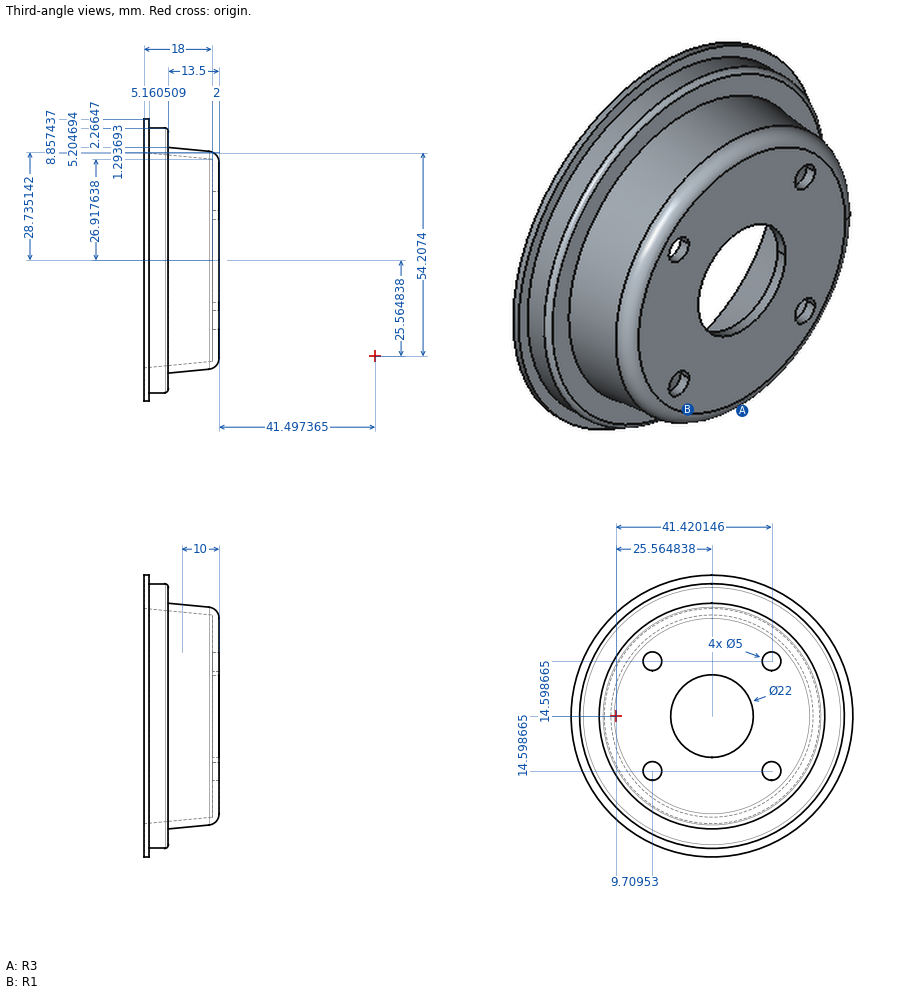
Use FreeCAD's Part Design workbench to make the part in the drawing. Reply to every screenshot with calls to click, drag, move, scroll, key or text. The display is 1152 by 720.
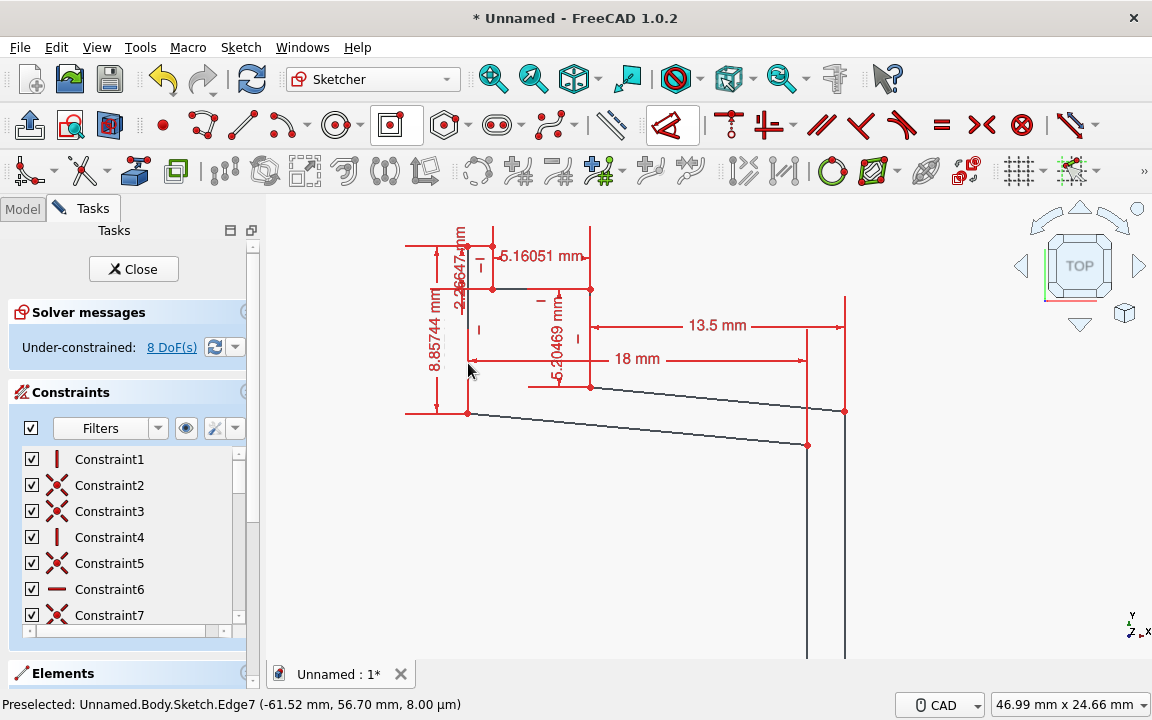
scroll(507, 292, down, 7)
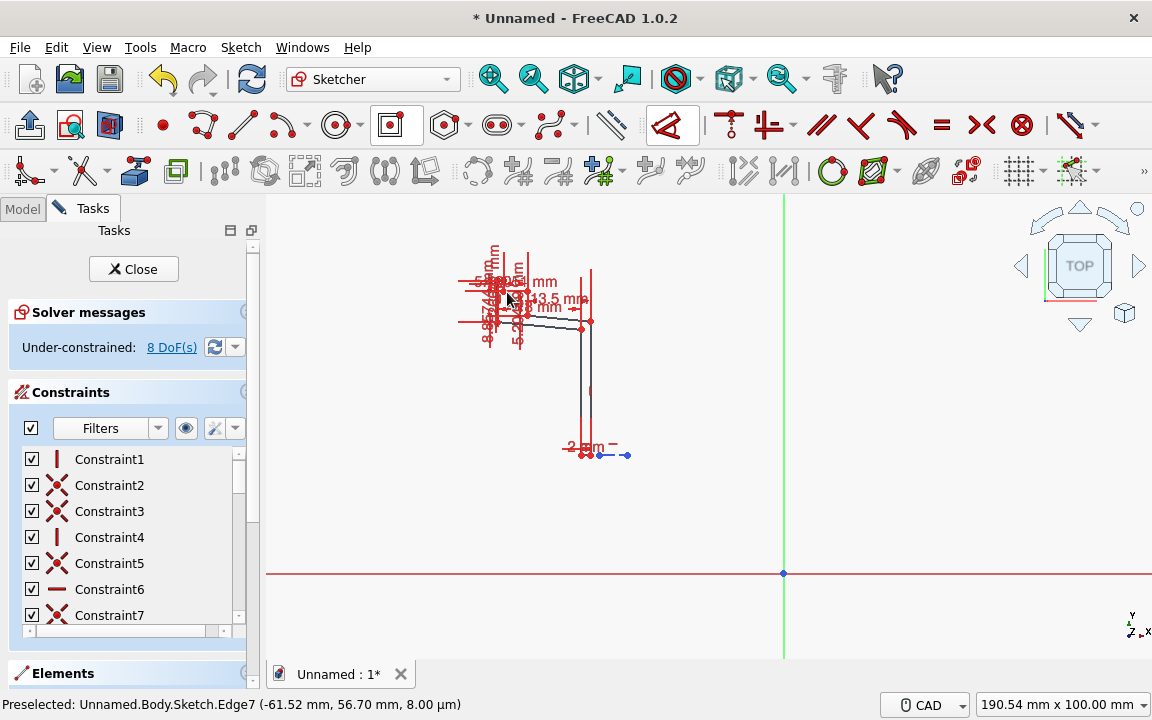
click(498, 322)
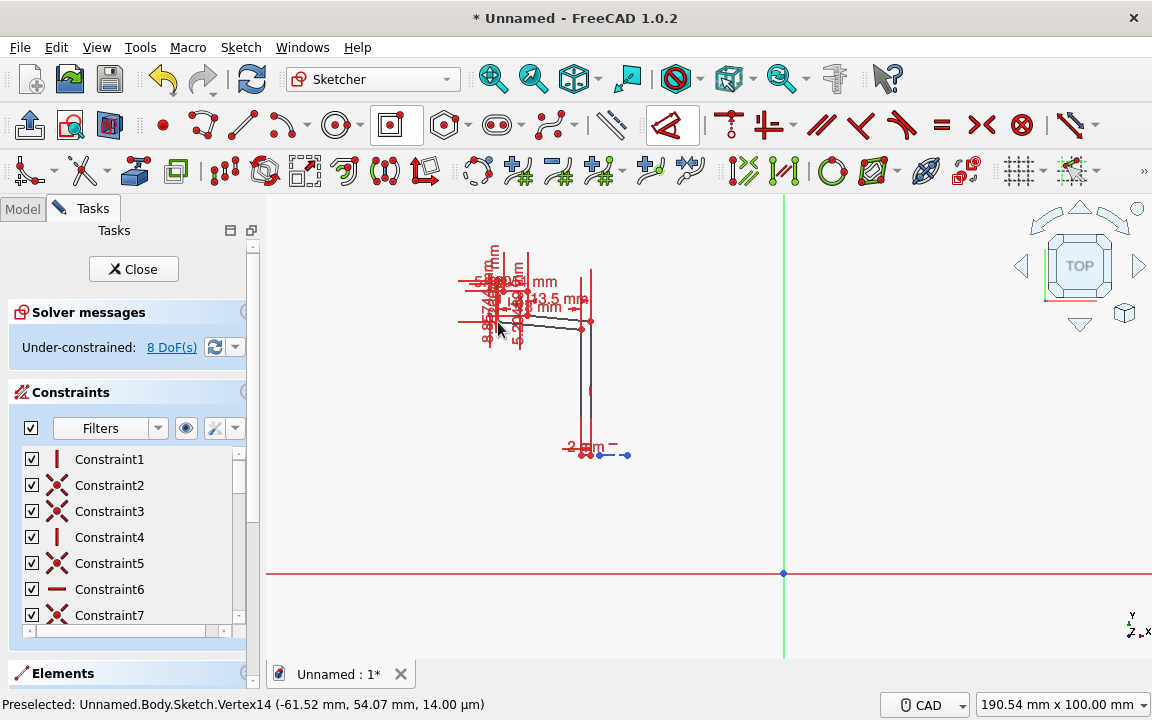
key(i)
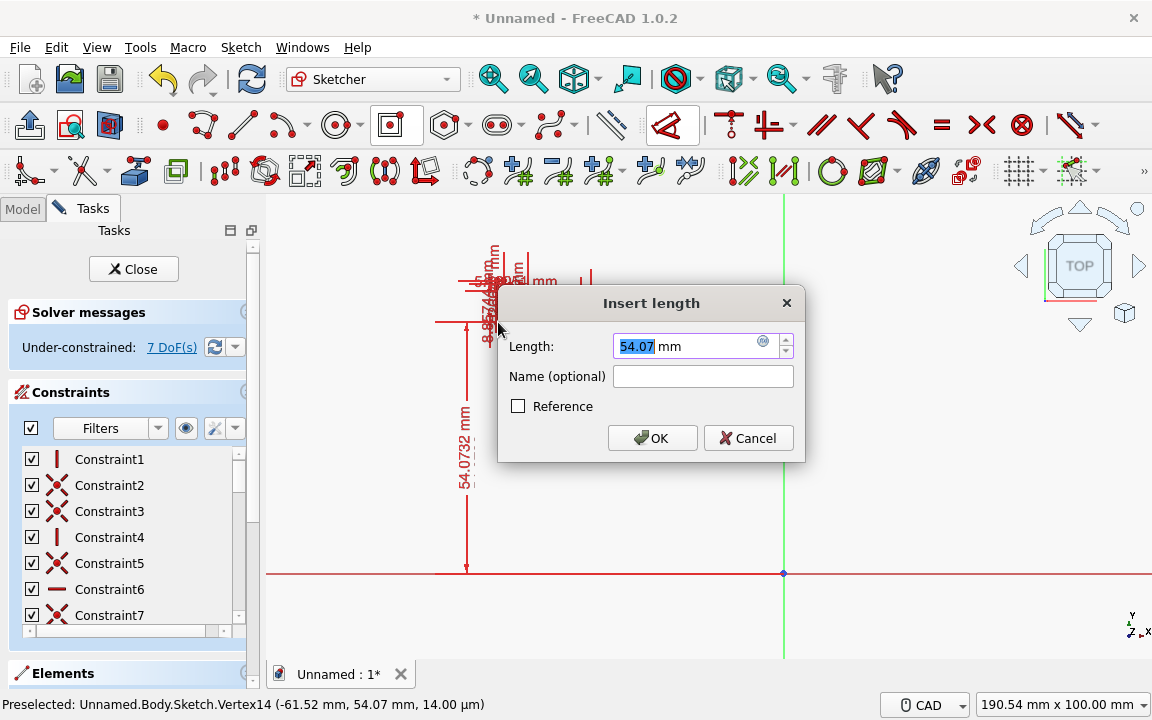
text(54.2074)
key(Return)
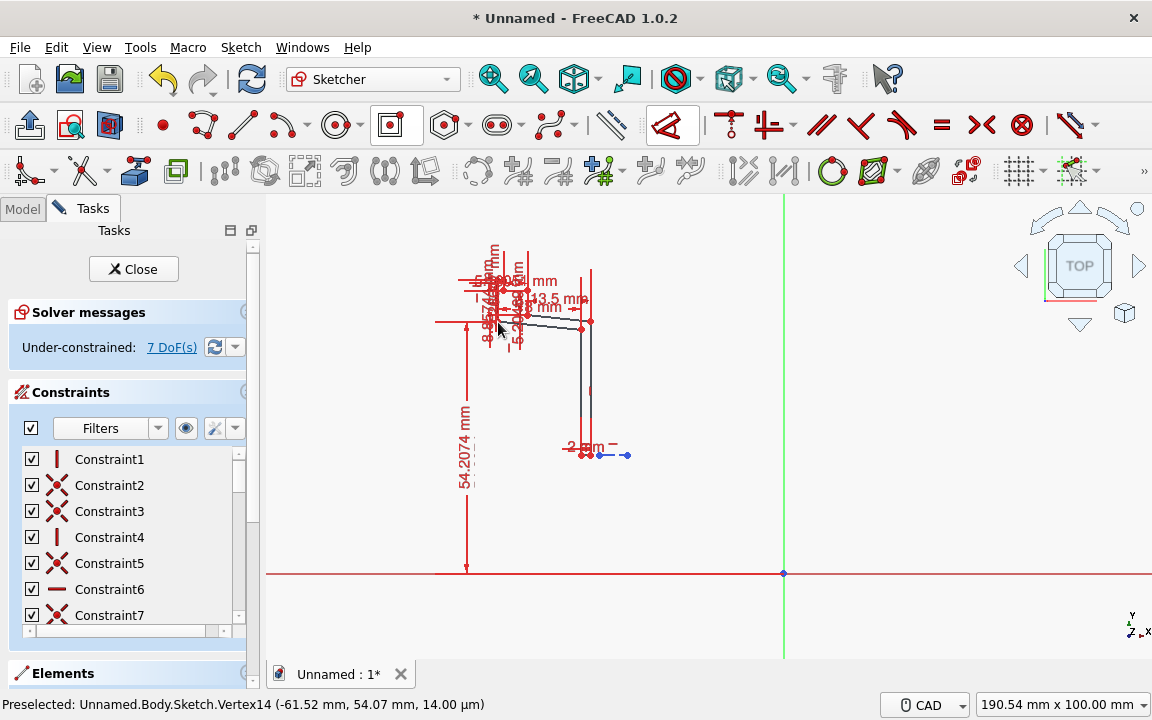
scroll(591, 415, up, 2)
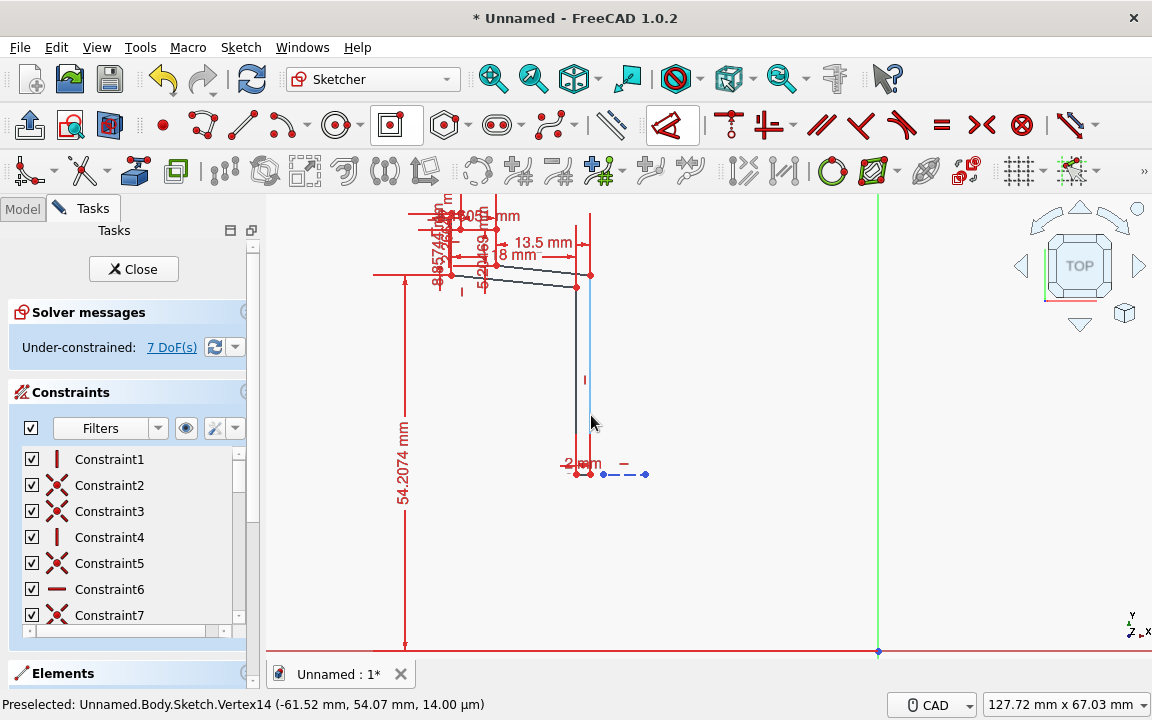
click(590, 415)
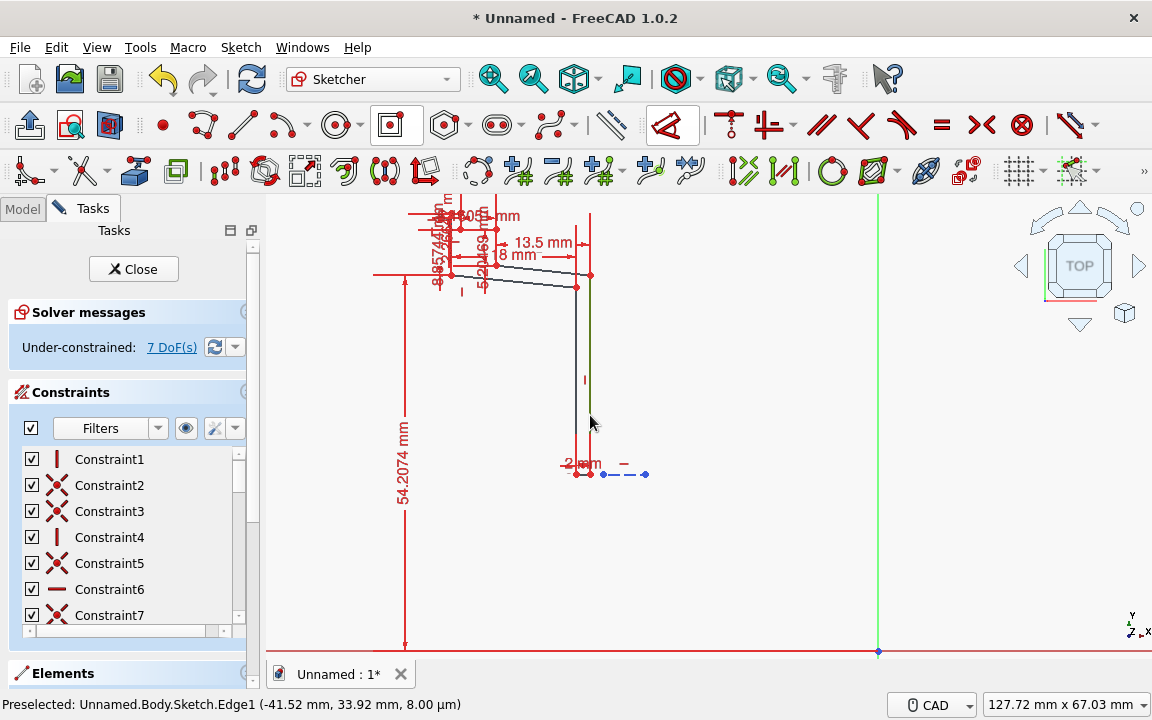
key(i)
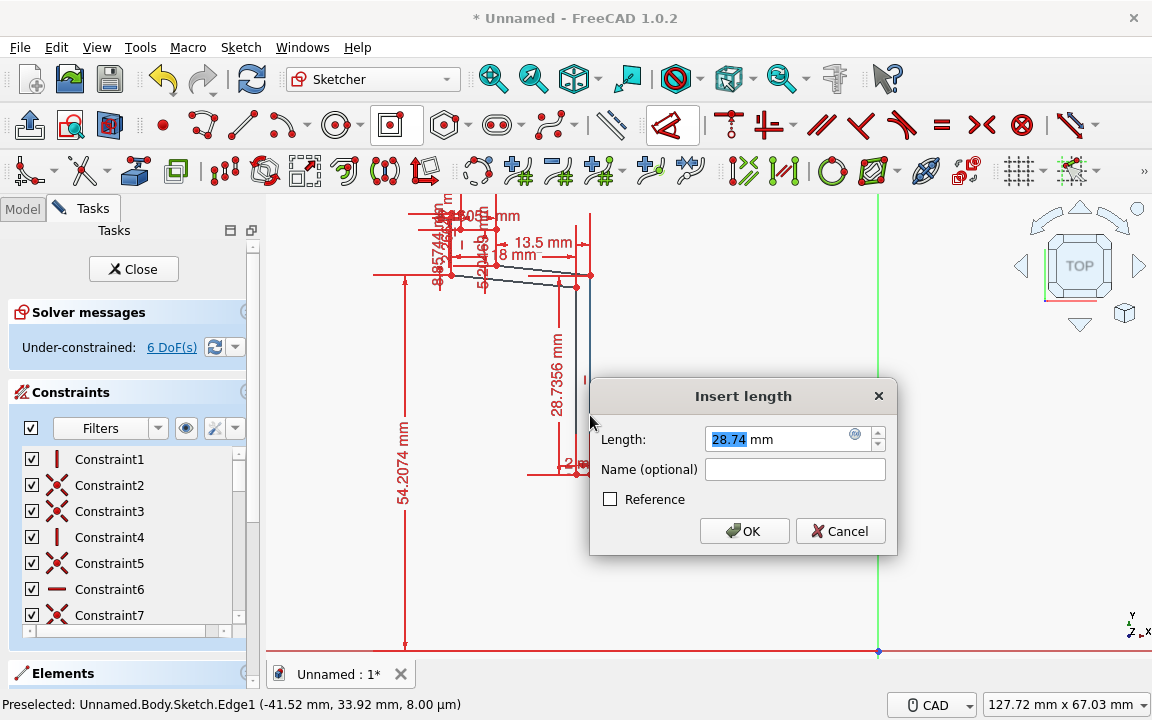
text(28.735142)
key(Return)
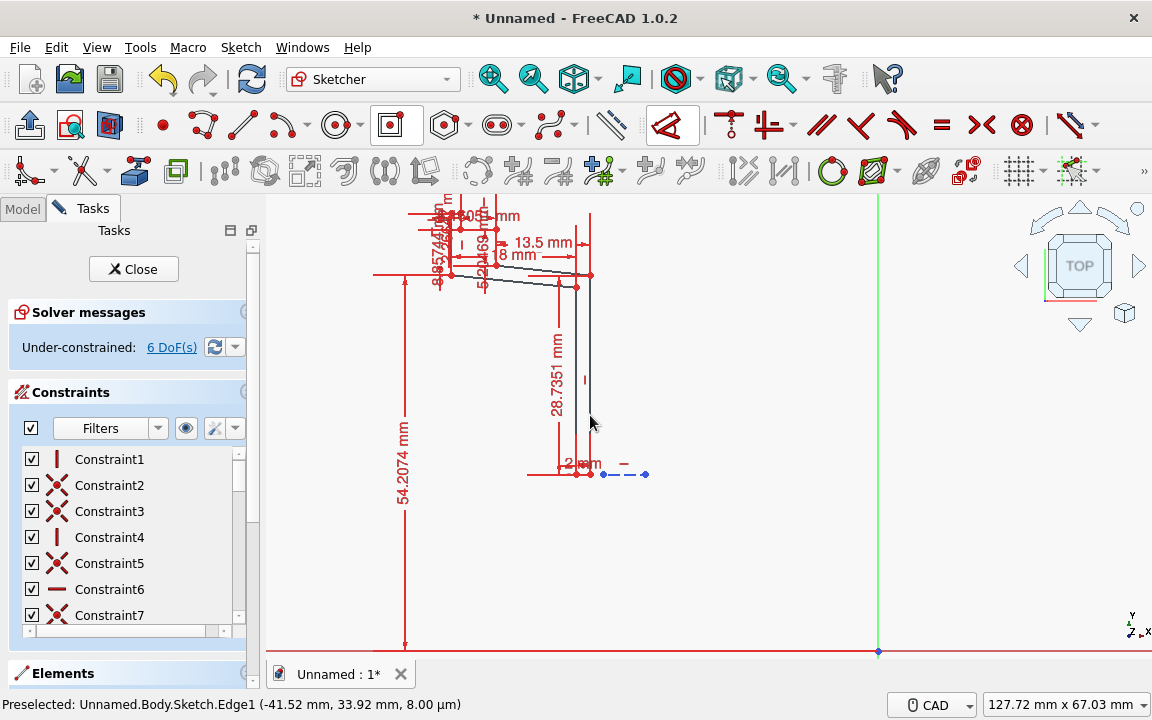
click(576, 344)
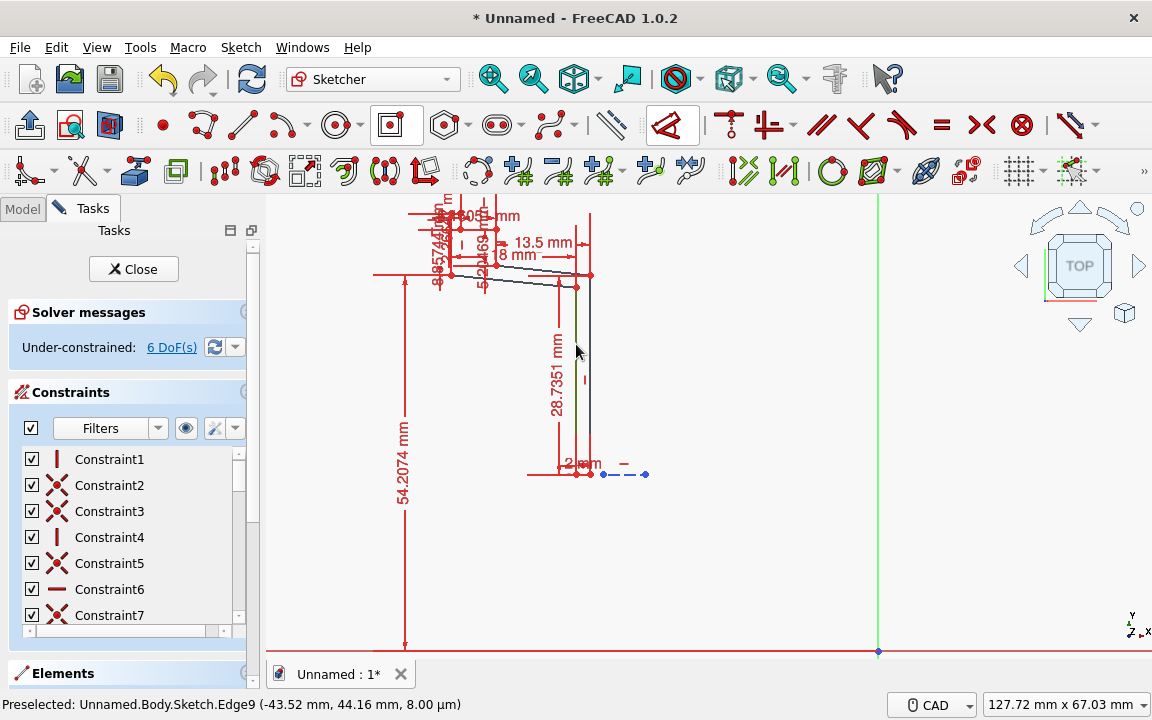
key(i)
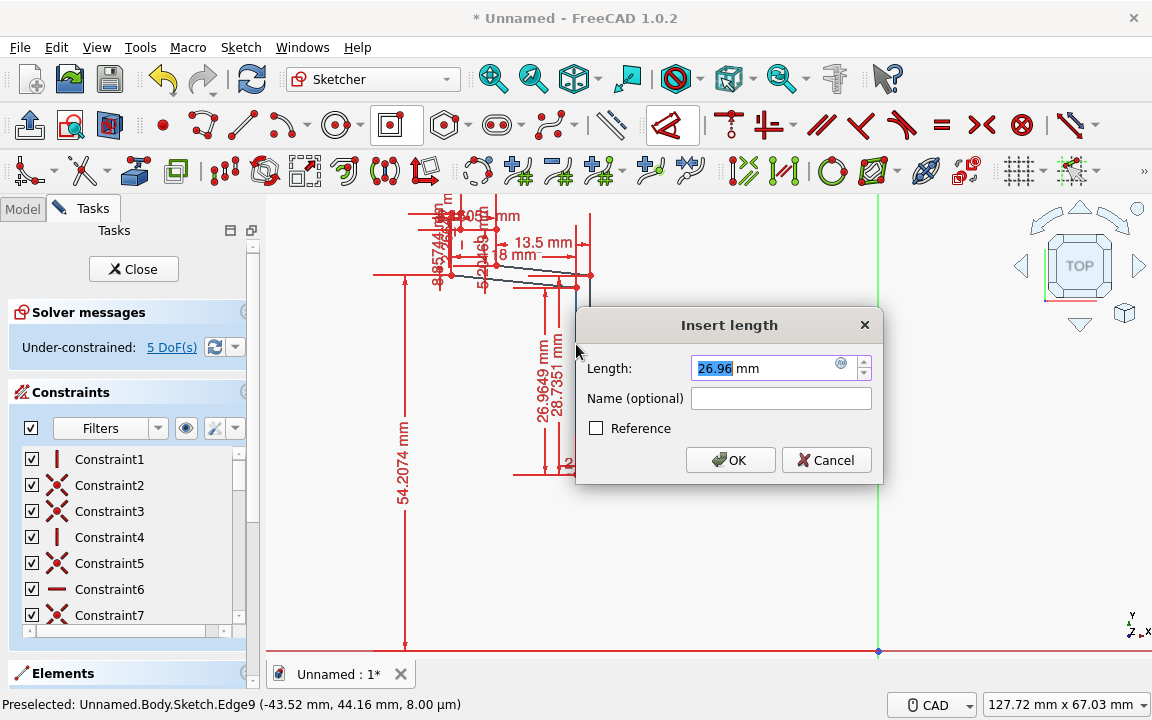
text(26.917638)
key(Return)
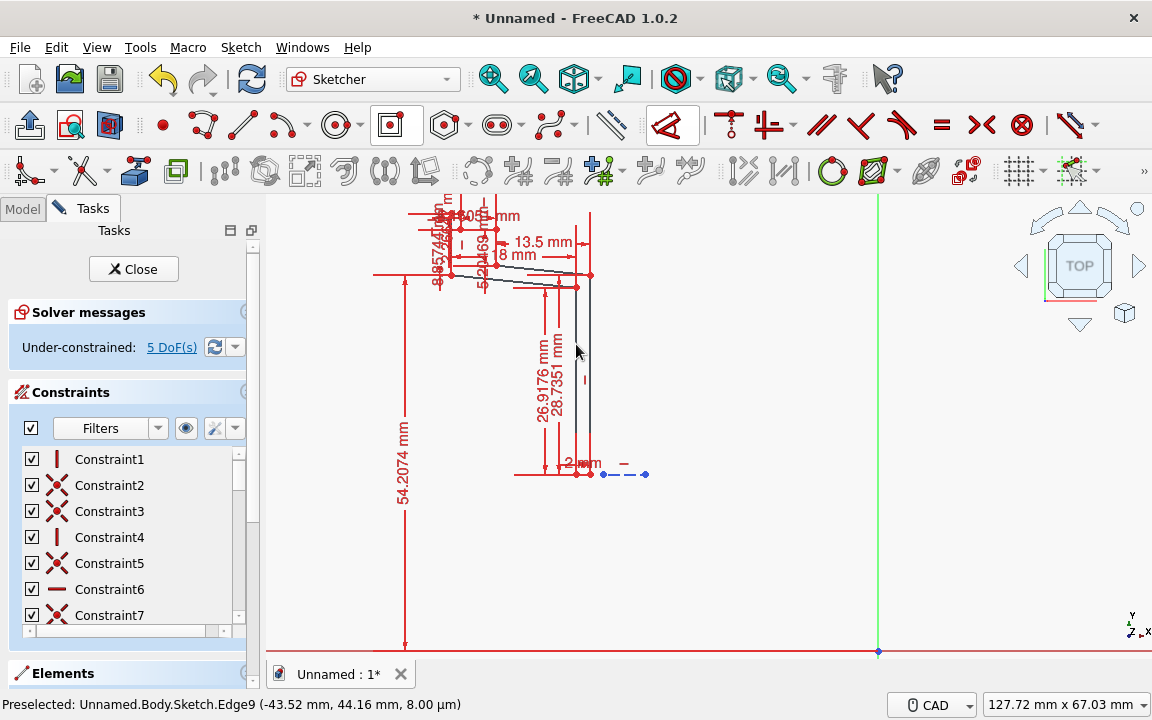
scroll(562, 272, up, 8)